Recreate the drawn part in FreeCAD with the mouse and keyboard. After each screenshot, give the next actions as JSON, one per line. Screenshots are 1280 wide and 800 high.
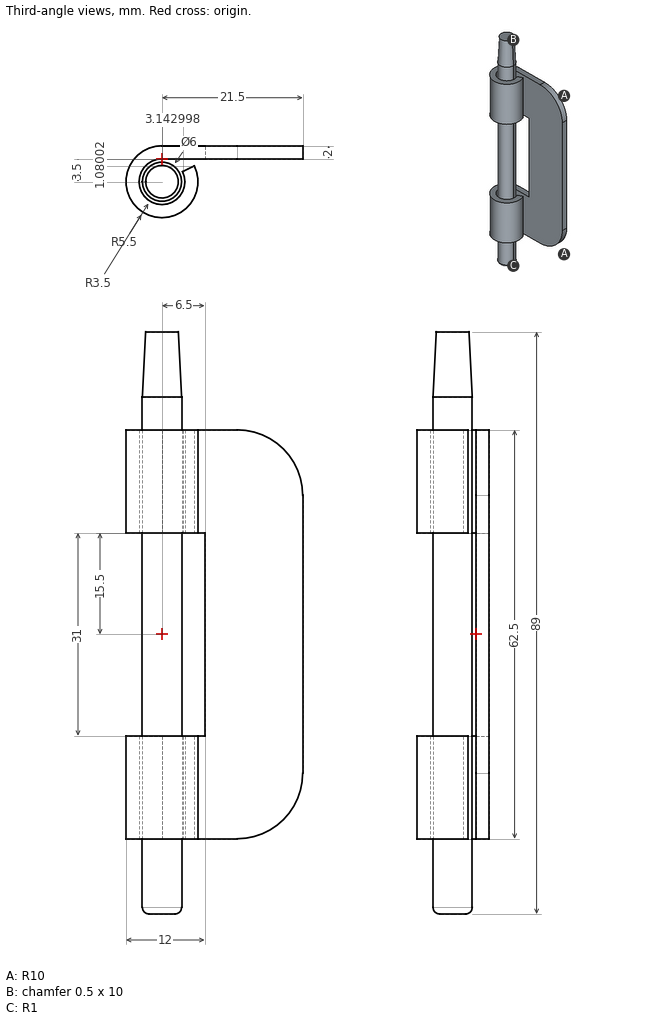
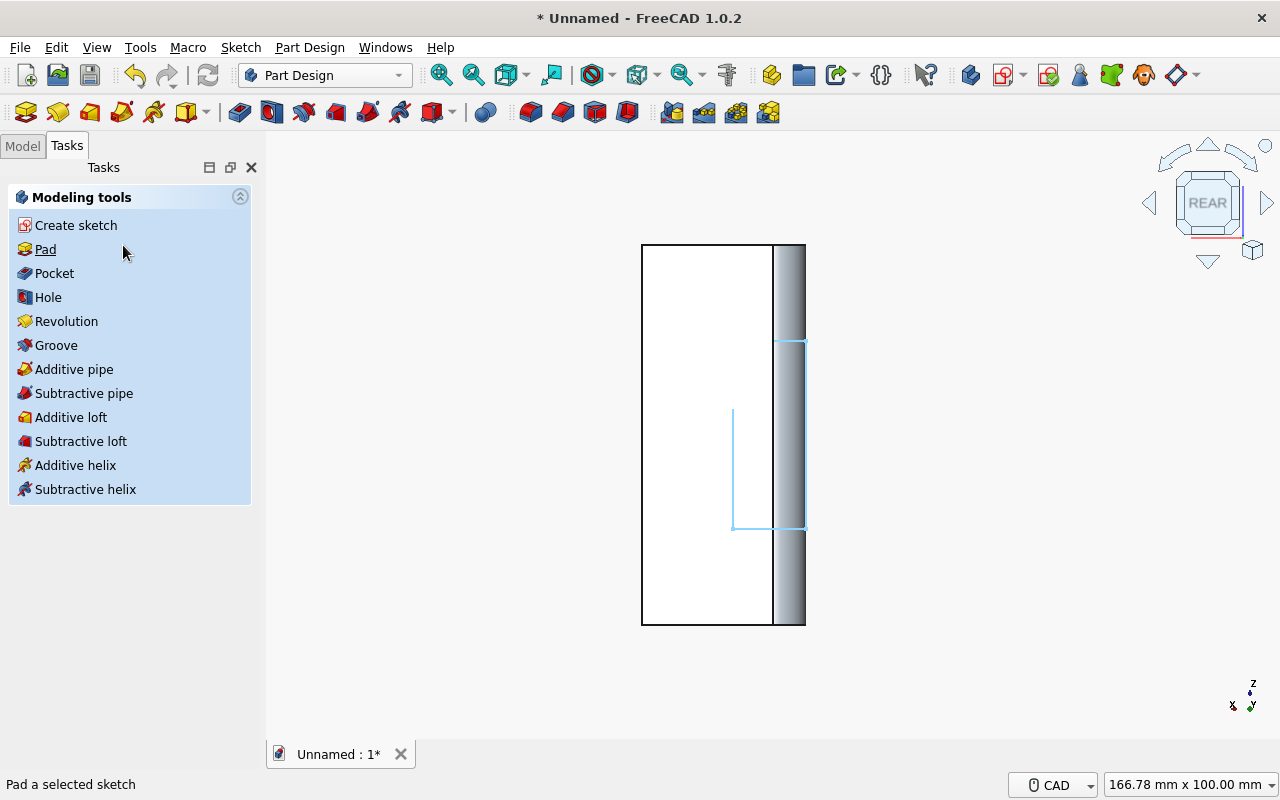
{"action": "left_click", "coordinate": [240, 112]}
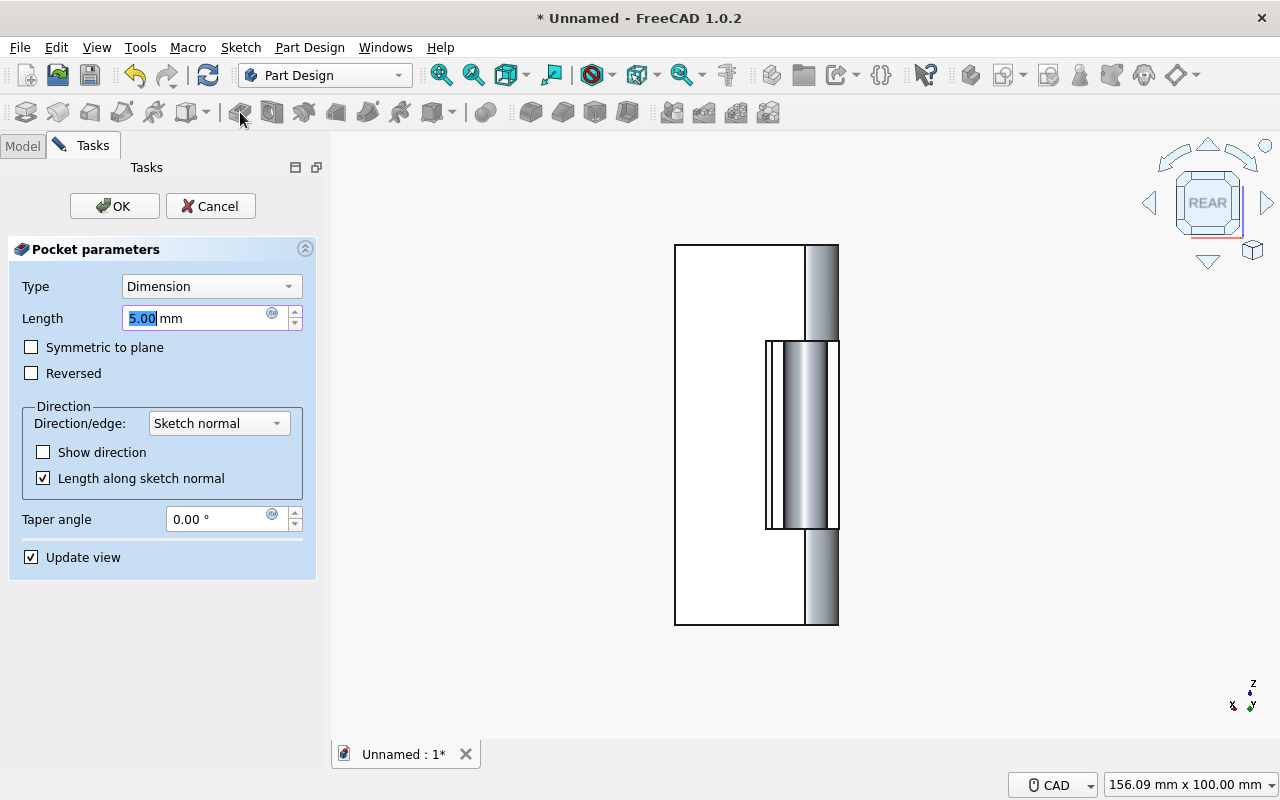
{"action": "left_click", "coordinate": [212, 286]}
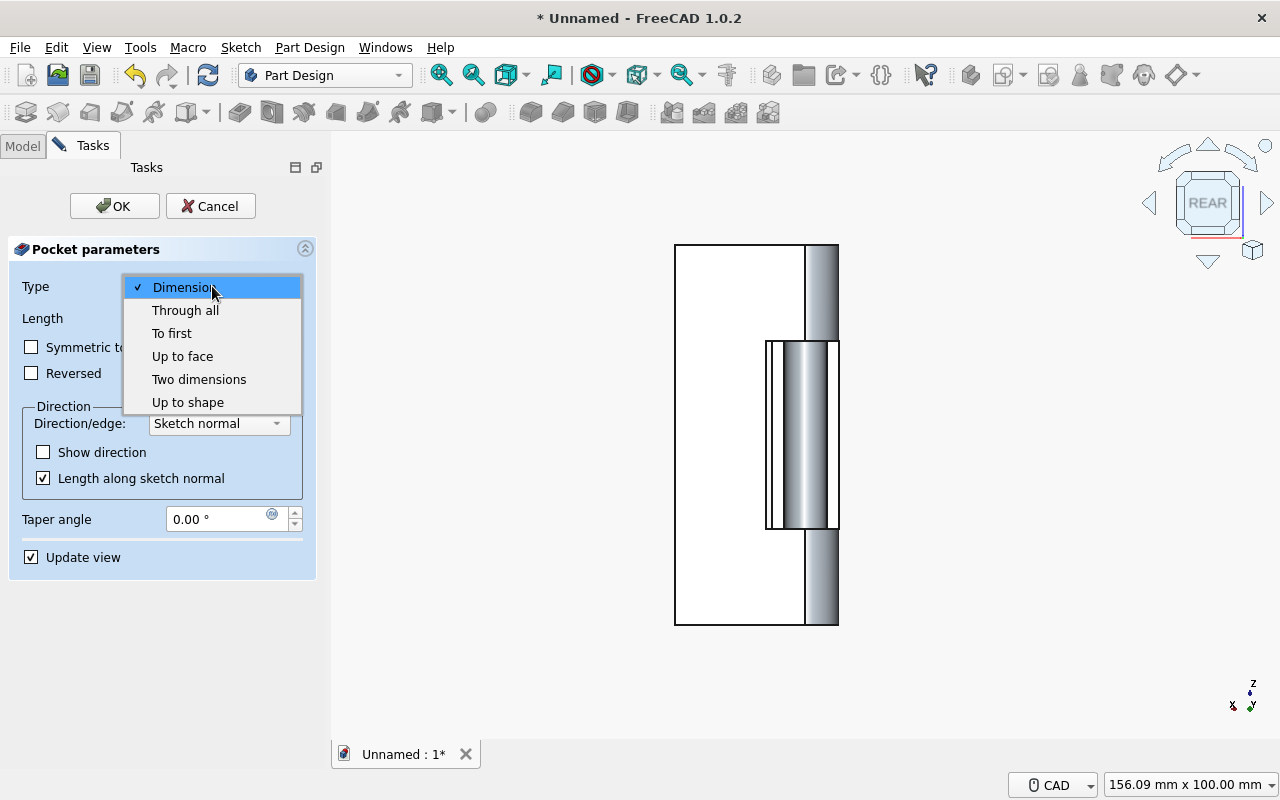
{"action": "left_click", "coordinate": [212, 310]}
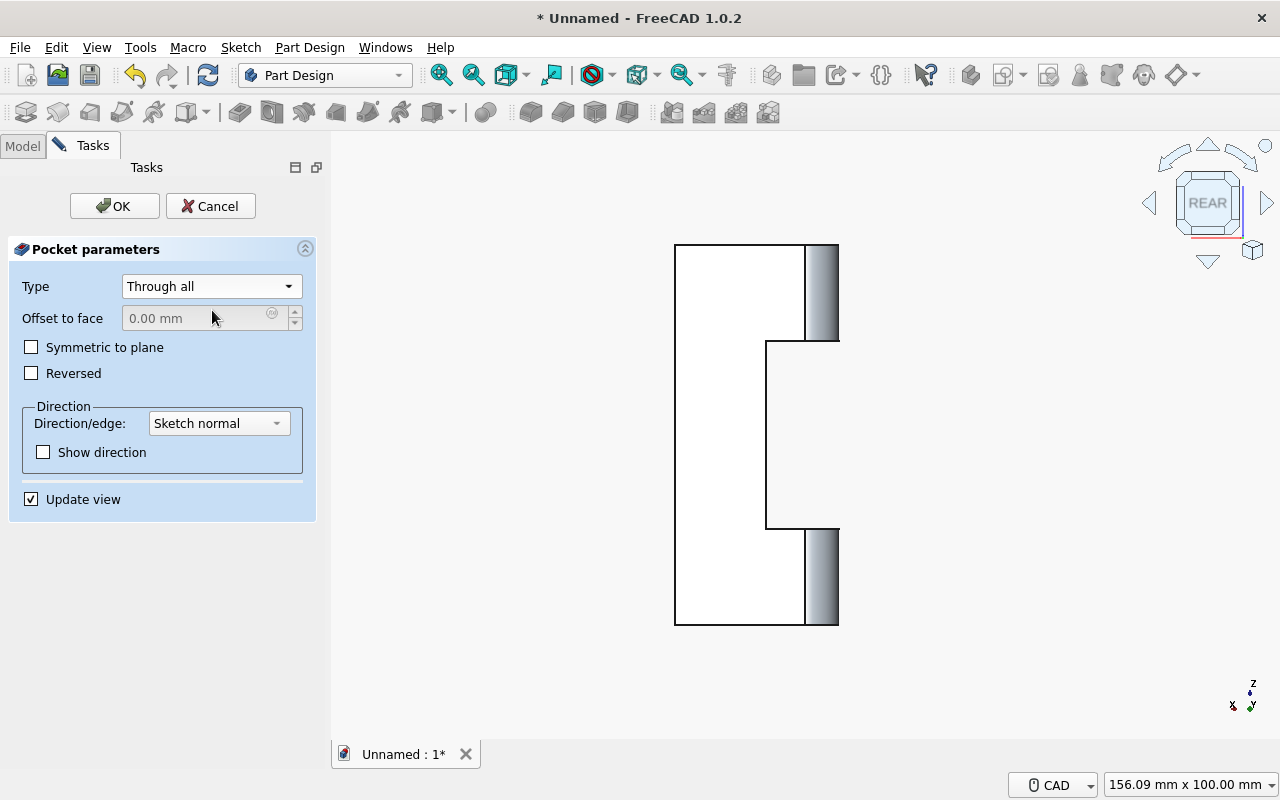
{"action": "left_click", "coordinate": [115, 206]}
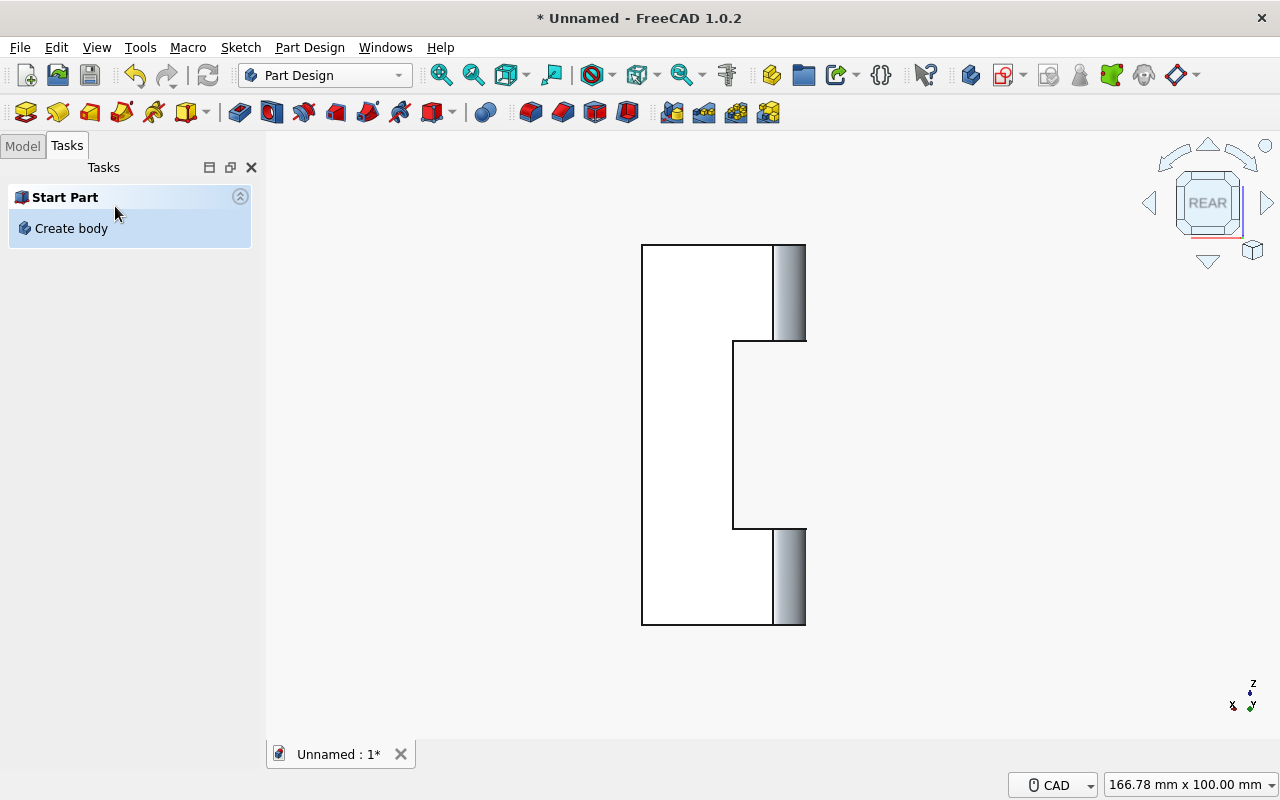
{"action": "scroll", "coordinate": [642, 244], "scroll_direction": "up", "scroll_amount": 6}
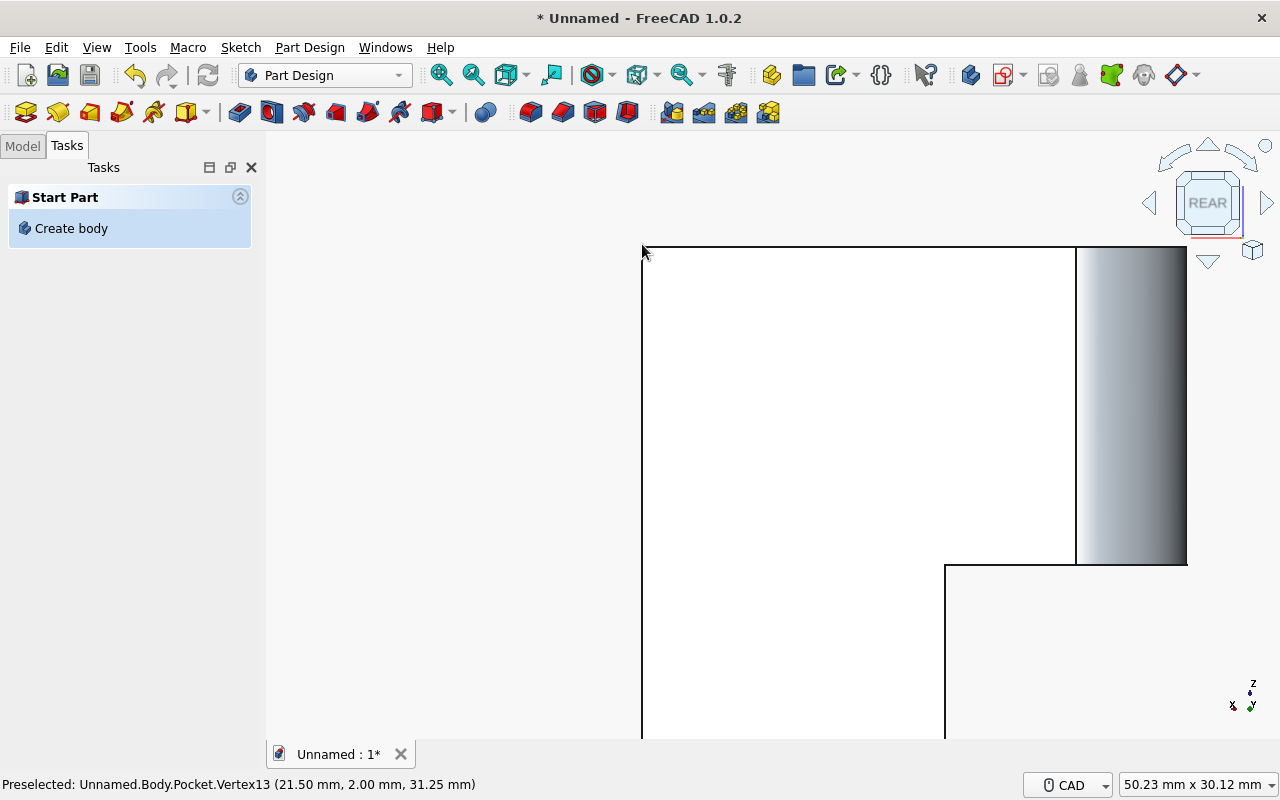
{"action": "key", "text": "v f"}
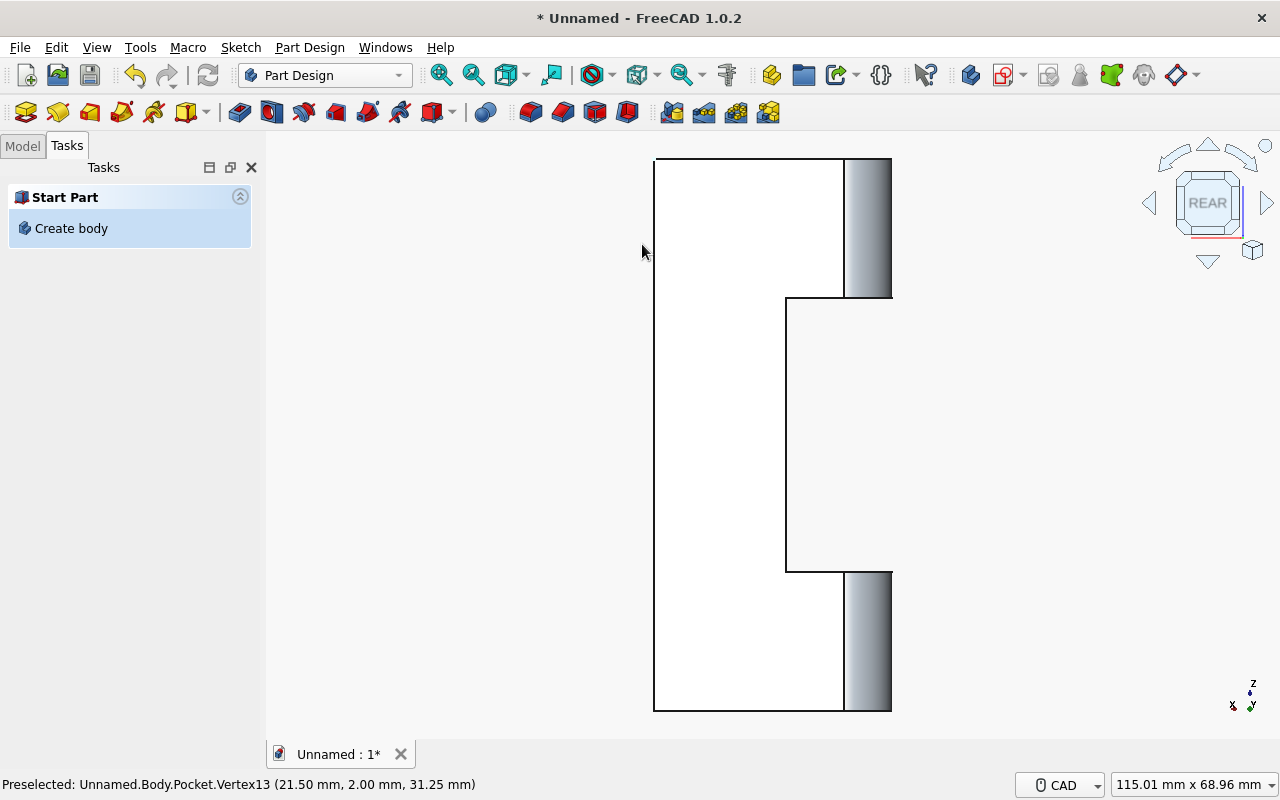
{"action": "key", "text": "0"}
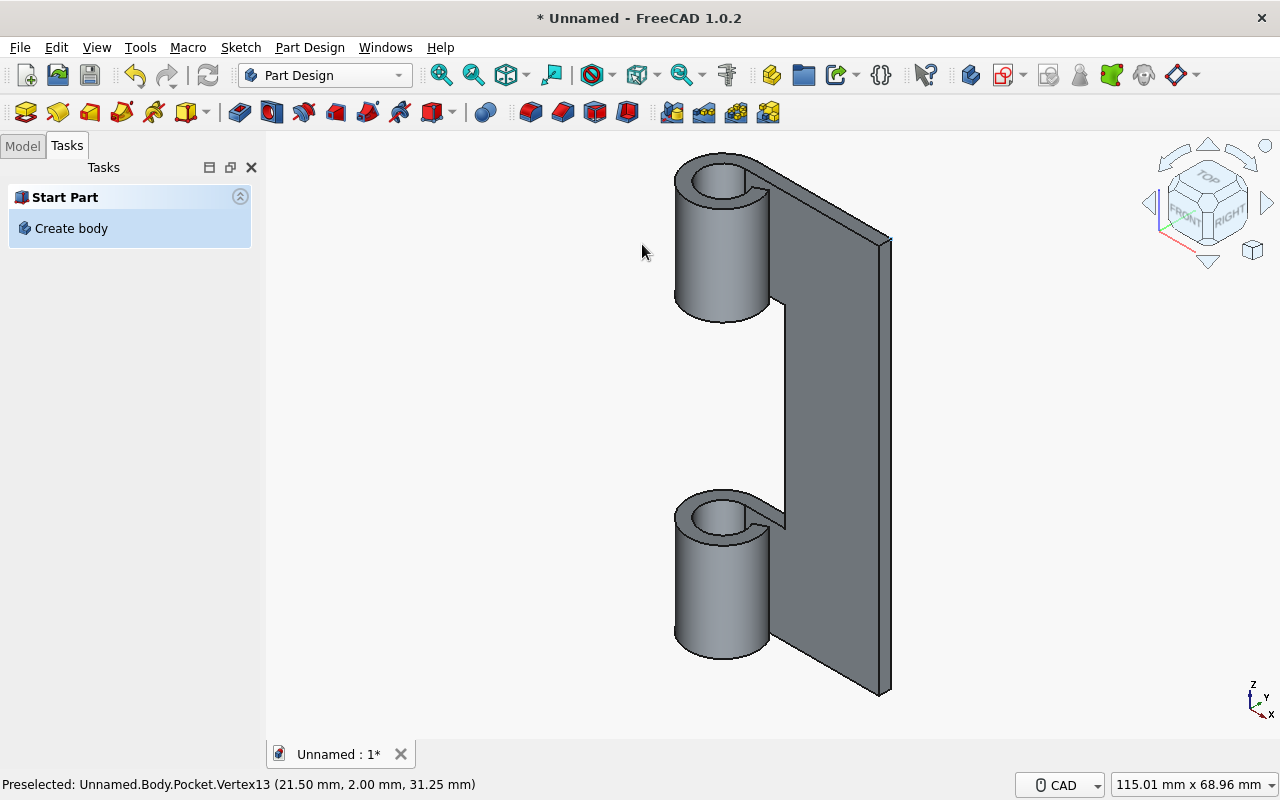
{"action": "left_click", "coordinate": [885, 241]}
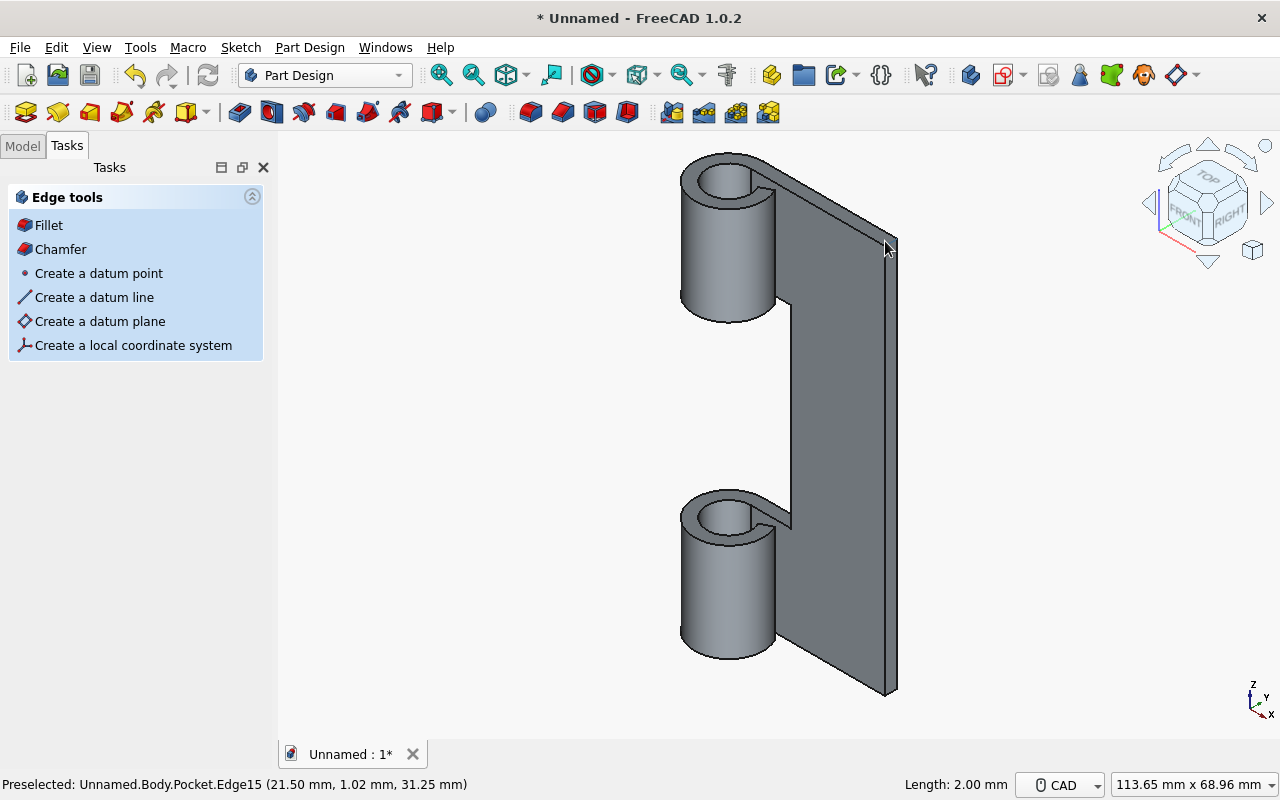
{"action": "scroll", "coordinate": [891, 691], "scroll_direction": "up", "scroll_amount": 5}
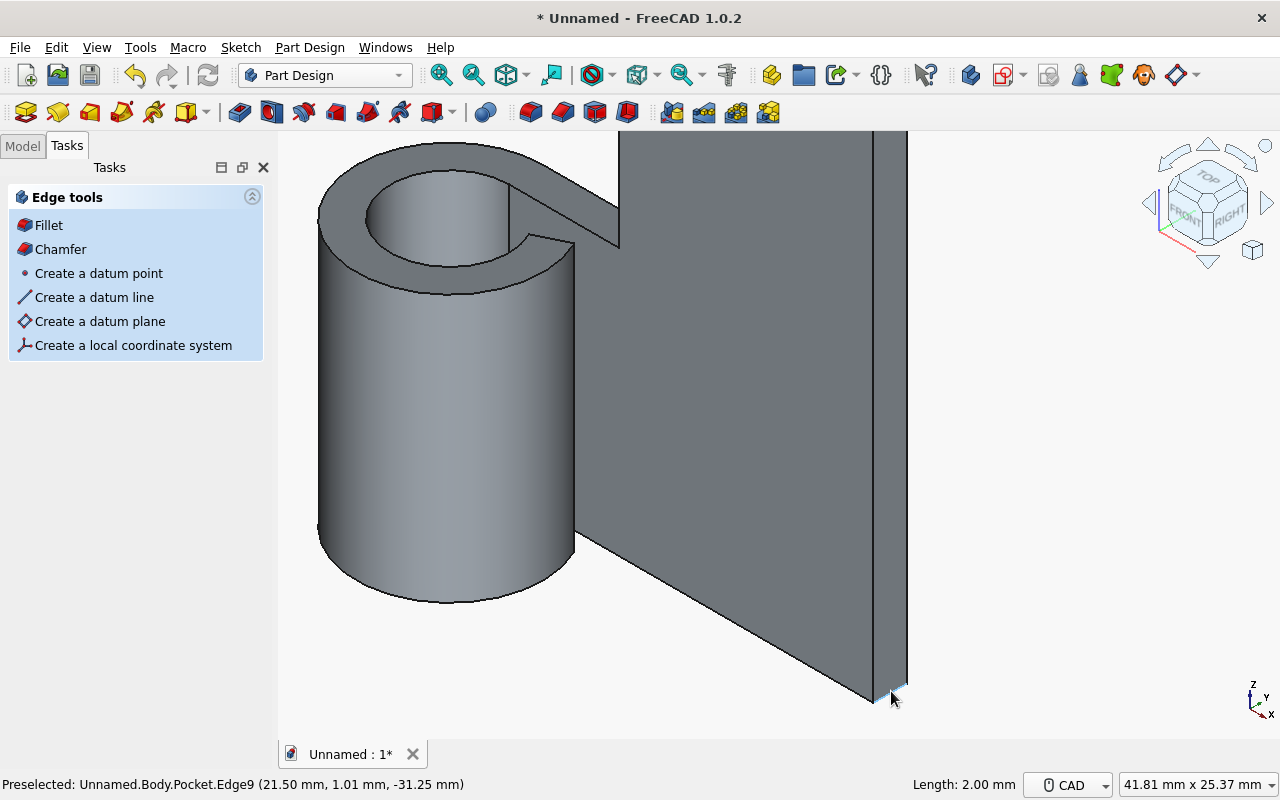
{"action": "key", "text": "v f"}